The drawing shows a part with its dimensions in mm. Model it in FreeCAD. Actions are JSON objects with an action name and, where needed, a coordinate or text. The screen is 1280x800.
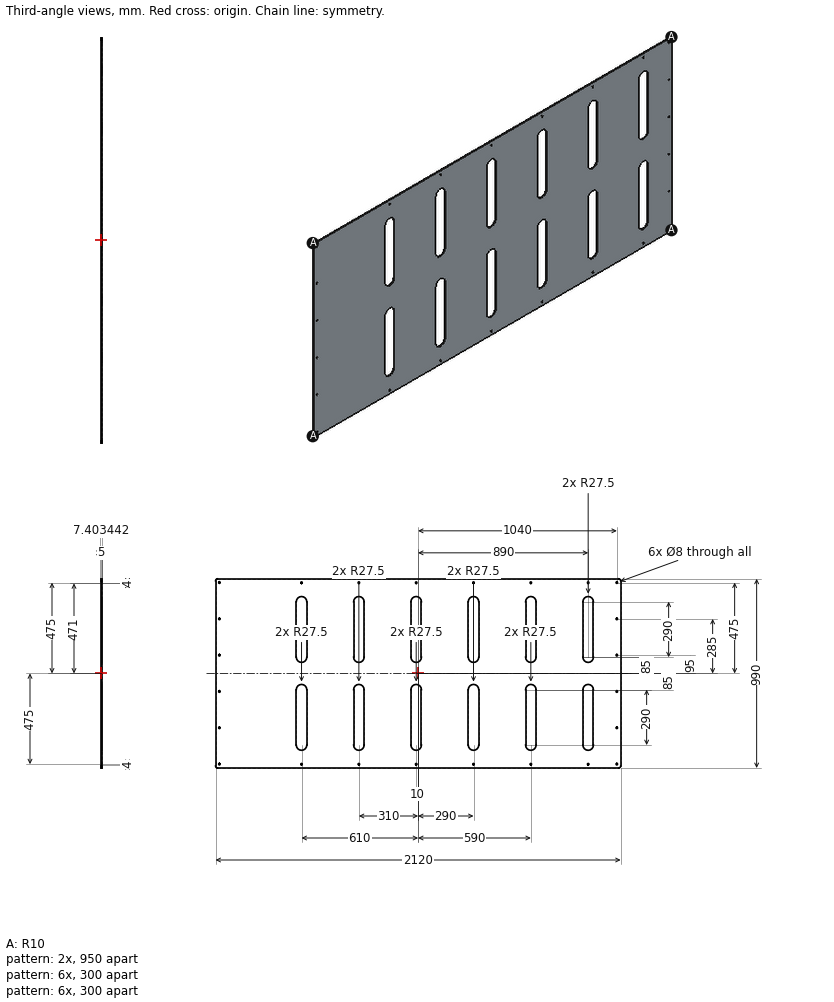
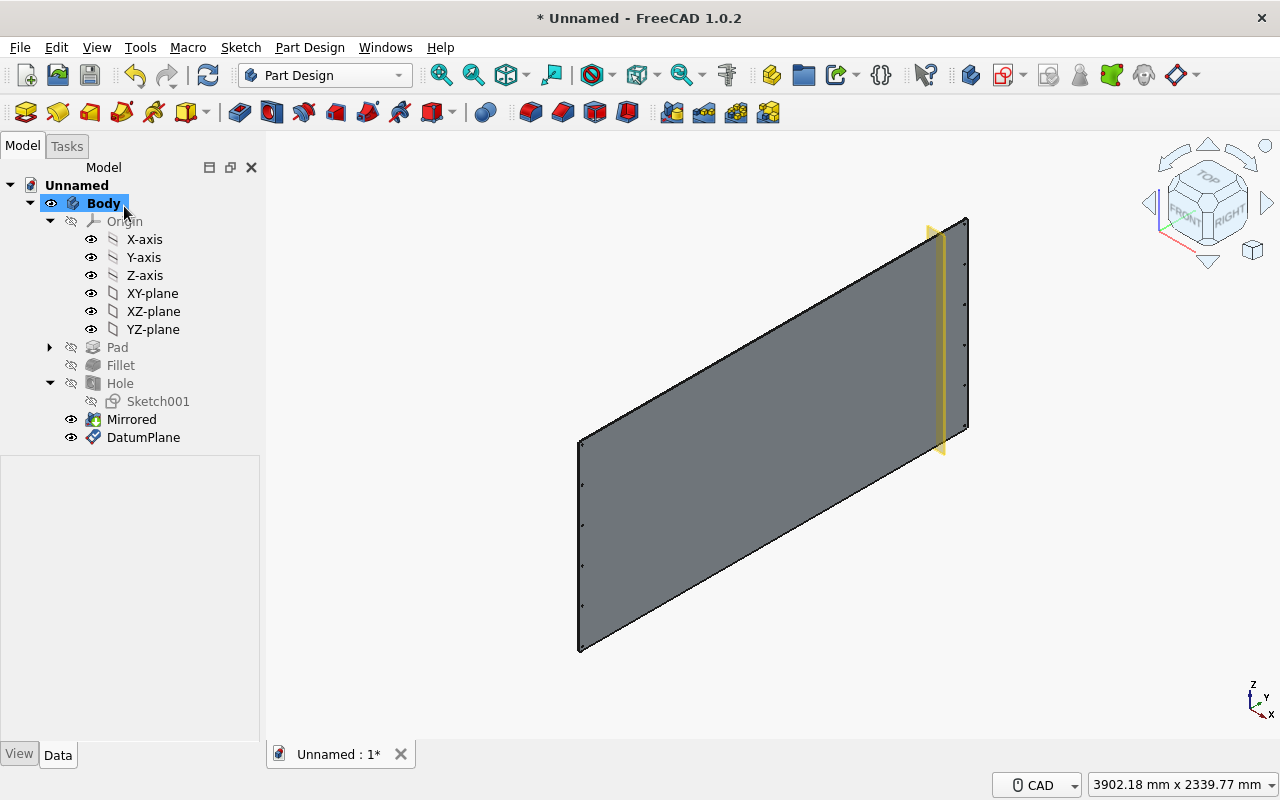
{"action": "left_click", "coordinate": [116, 437]}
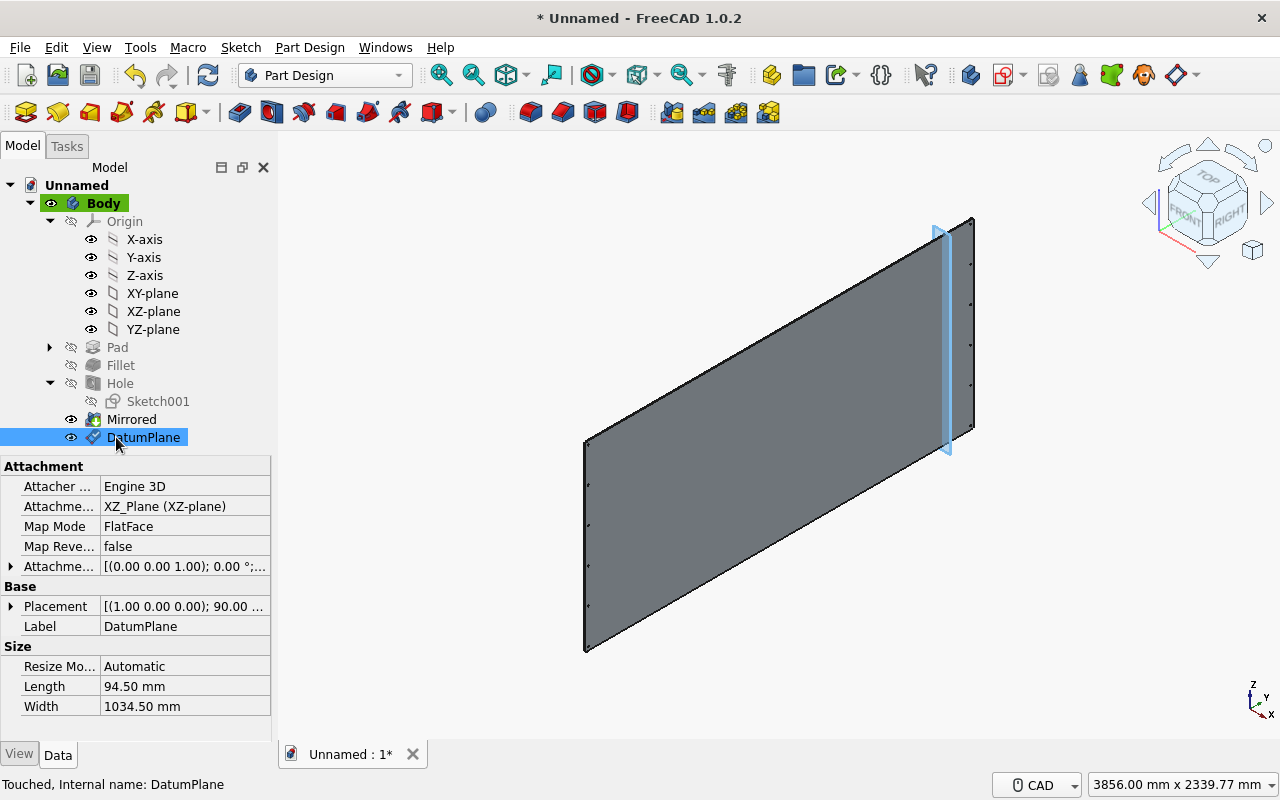
{"action": "left_click", "coordinate": [1004, 76]}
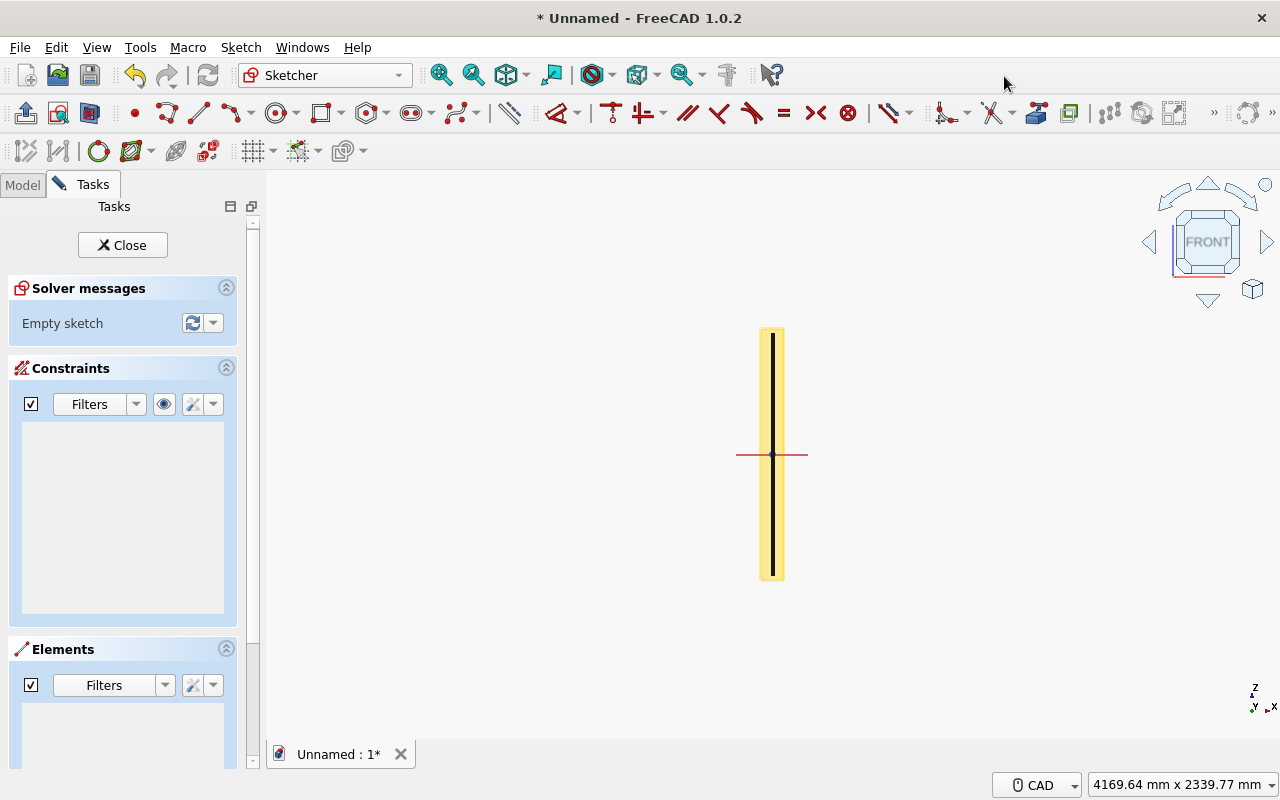
{"action": "left_click", "coordinate": [90, 114]}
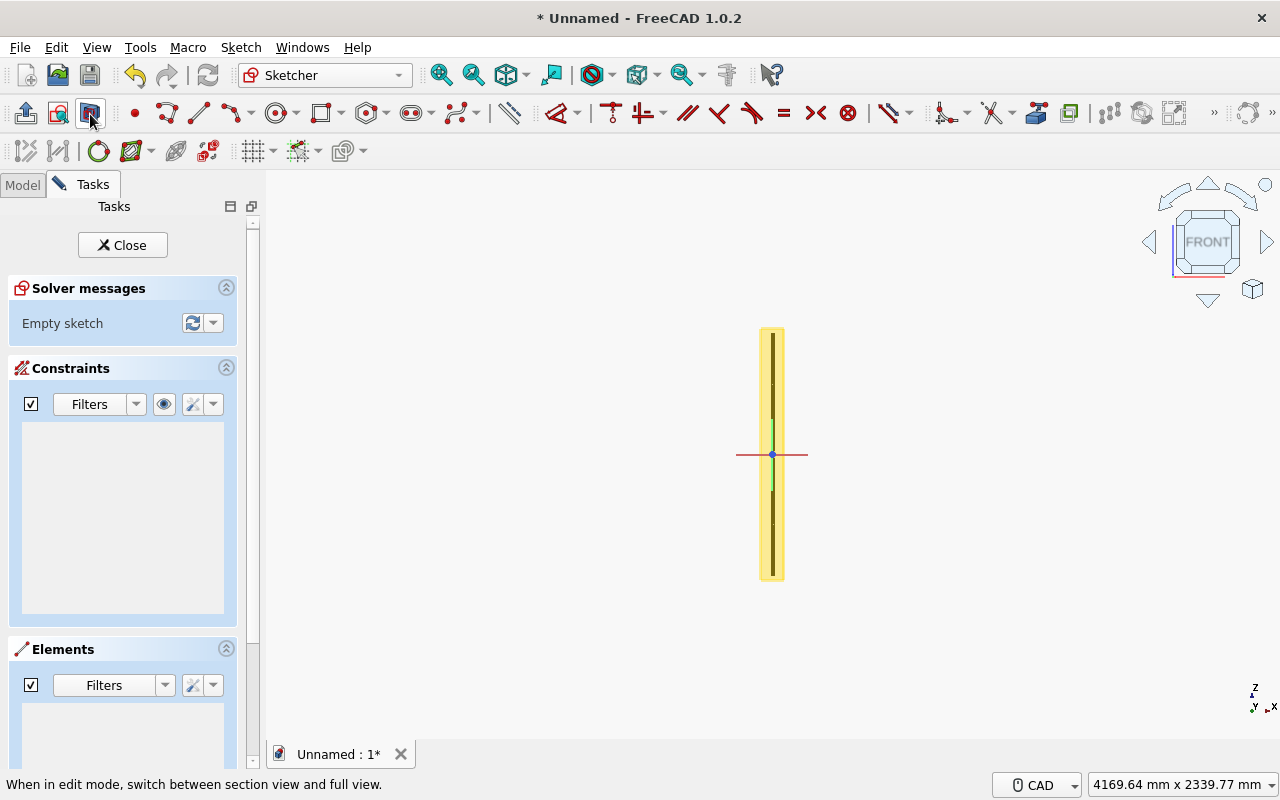
{"action": "scroll", "coordinate": [776, 333], "scroll_direction": "up", "scroll_amount": 15}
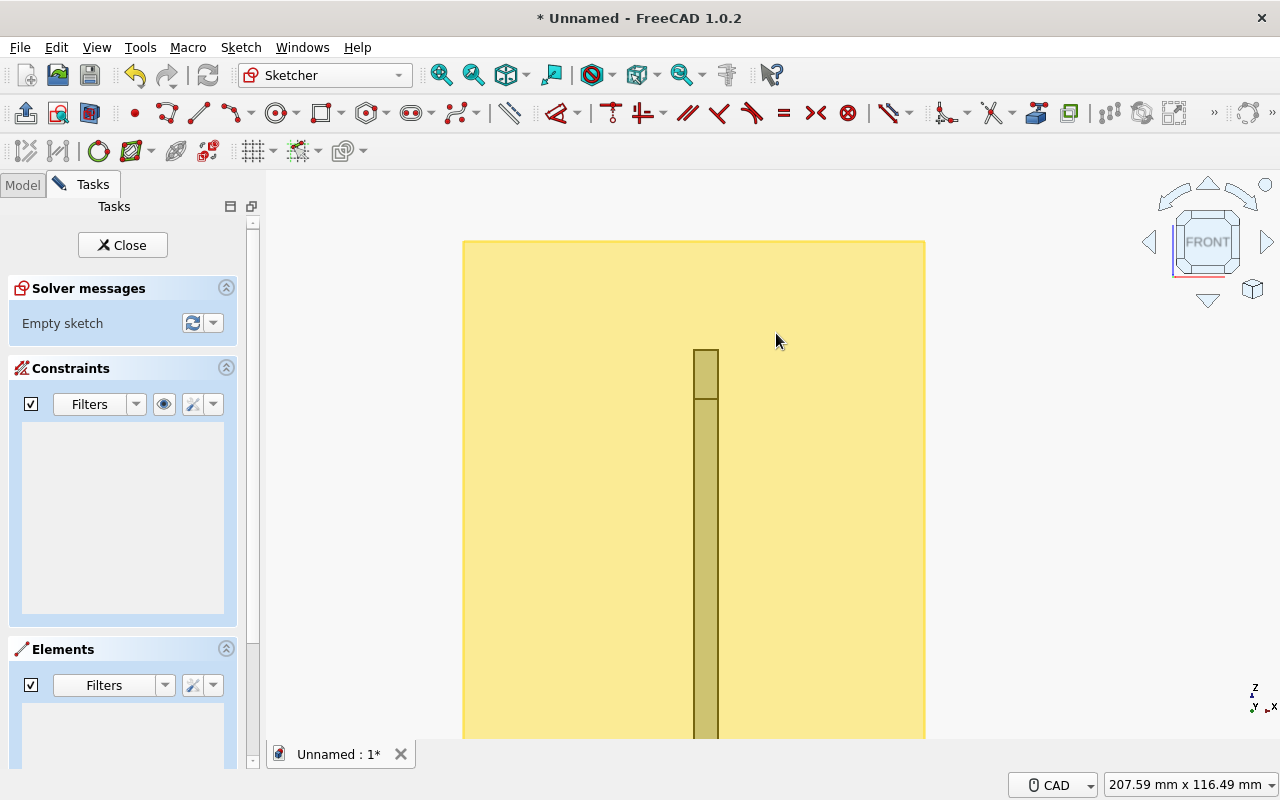
{"action": "scroll", "coordinate": [692, 458], "scroll_direction": "up", "scroll_amount": 12}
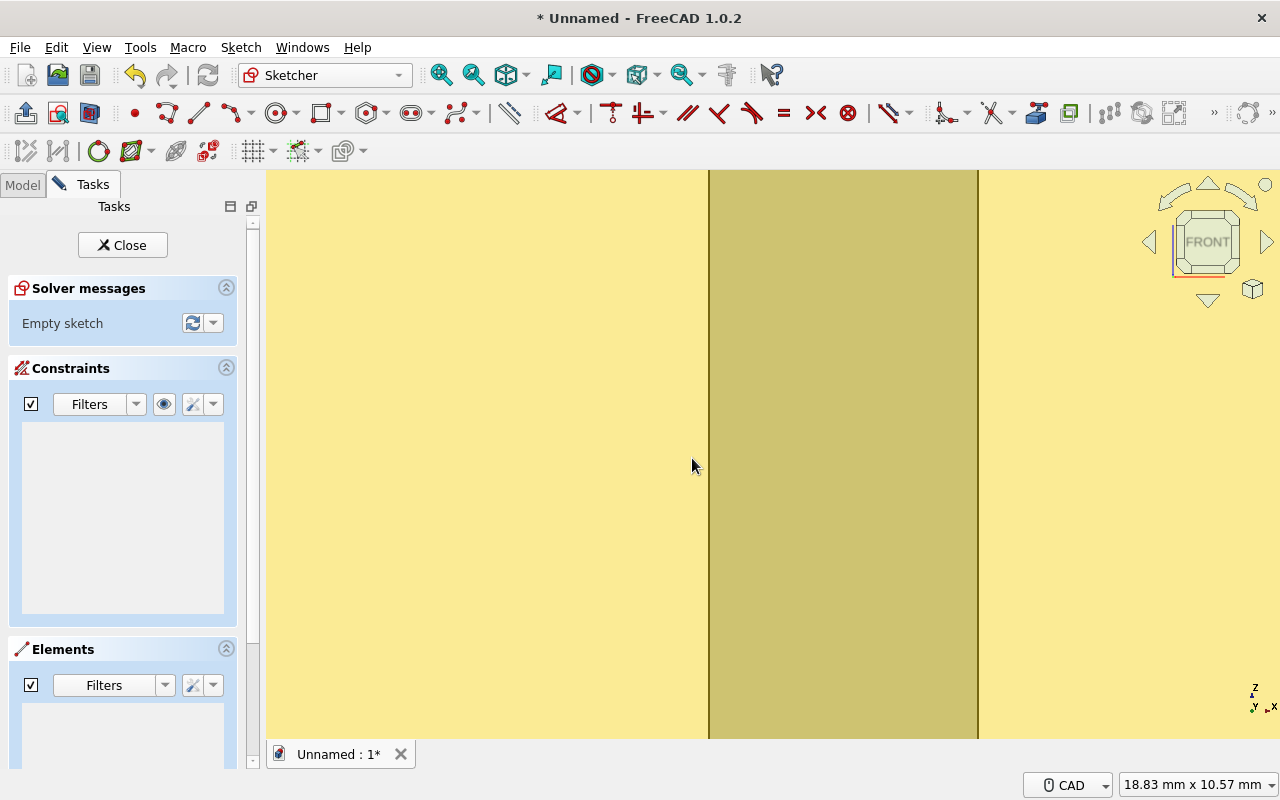
{"action": "left_click", "coordinate": [168, 114]}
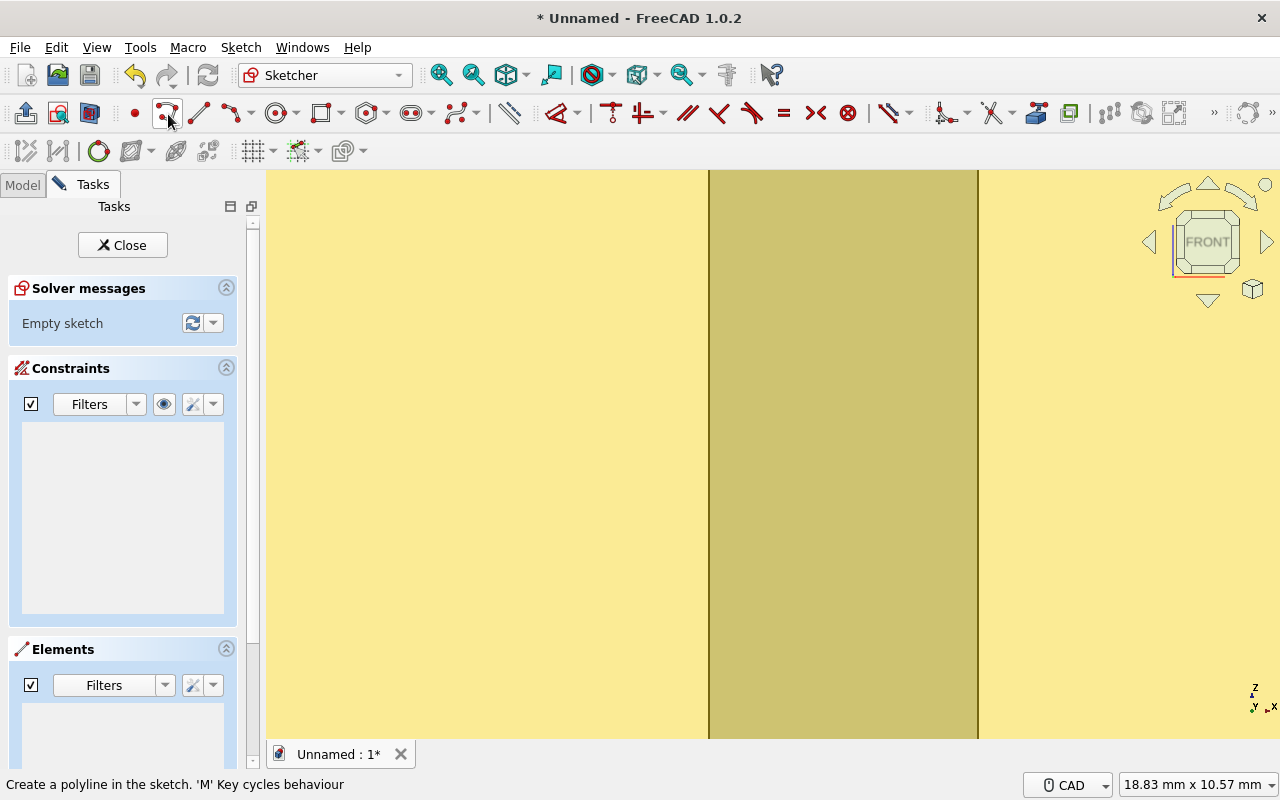
{"action": "left_click", "coordinate": [709, 555]}
{"action": "left_click", "coordinate": [580, 340]}
{"action": "left_click", "coordinate": [978, 340]}
{"action": "left_click", "coordinate": [978, 555]}
{"action": "left_click", "coordinate": [709, 556]}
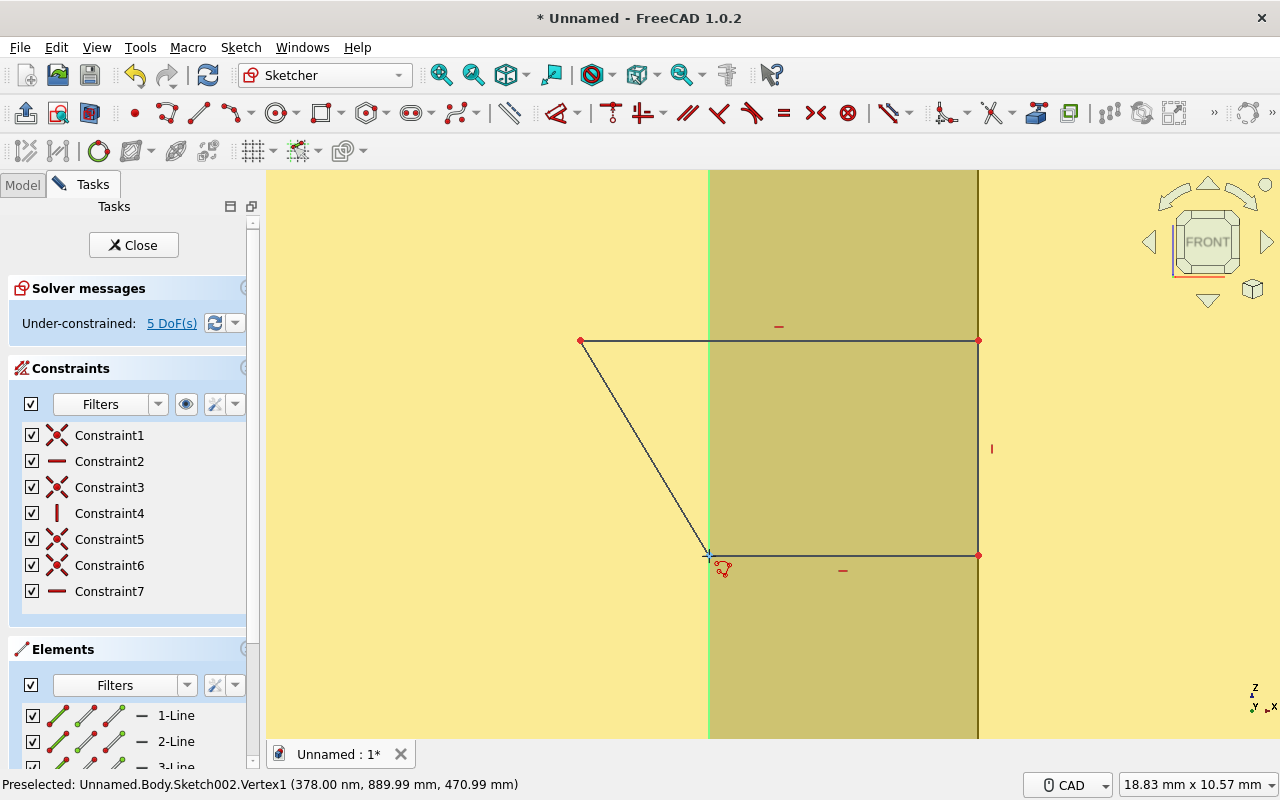
{"action": "left_click", "coordinate": [200, 114]}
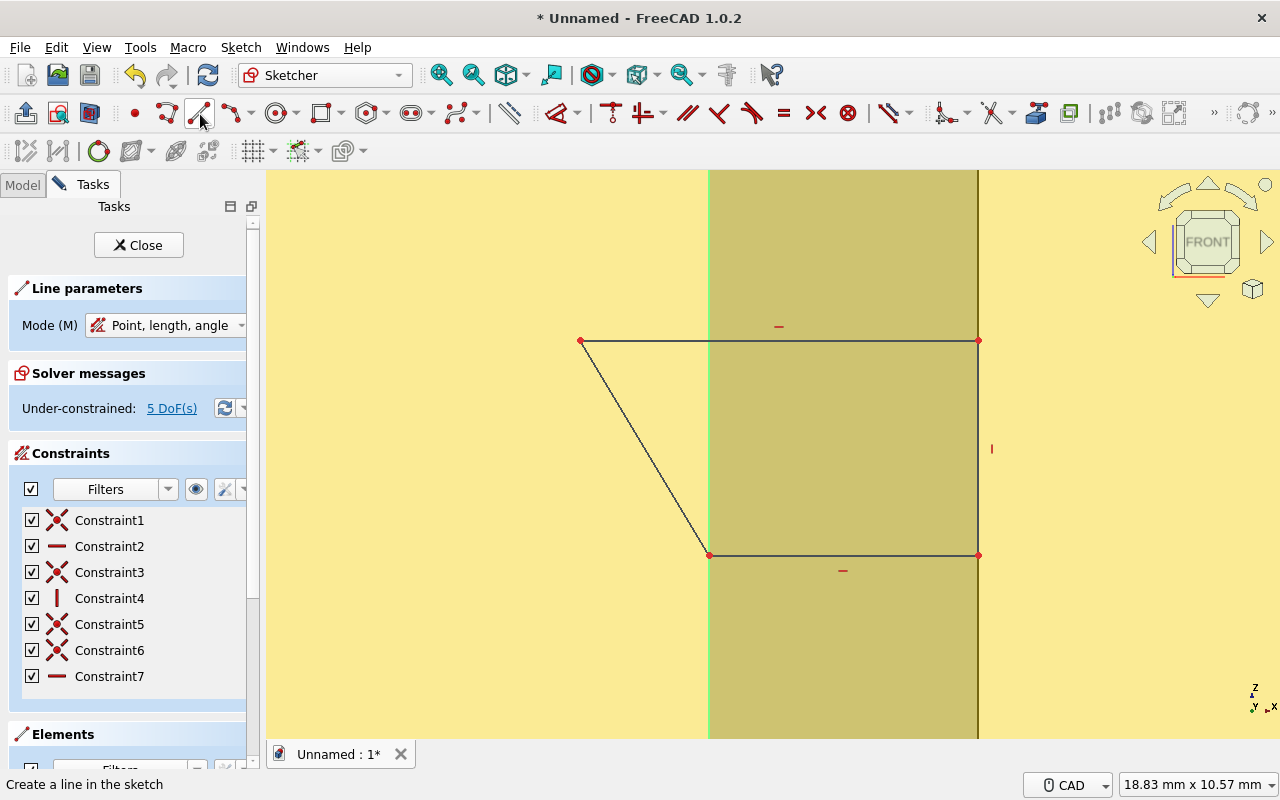
{"action": "left_click", "coordinate": [540, 340]}
{"action": "left_click", "coordinate": [420, 340]}
{"action": "key", "text": "Escape"}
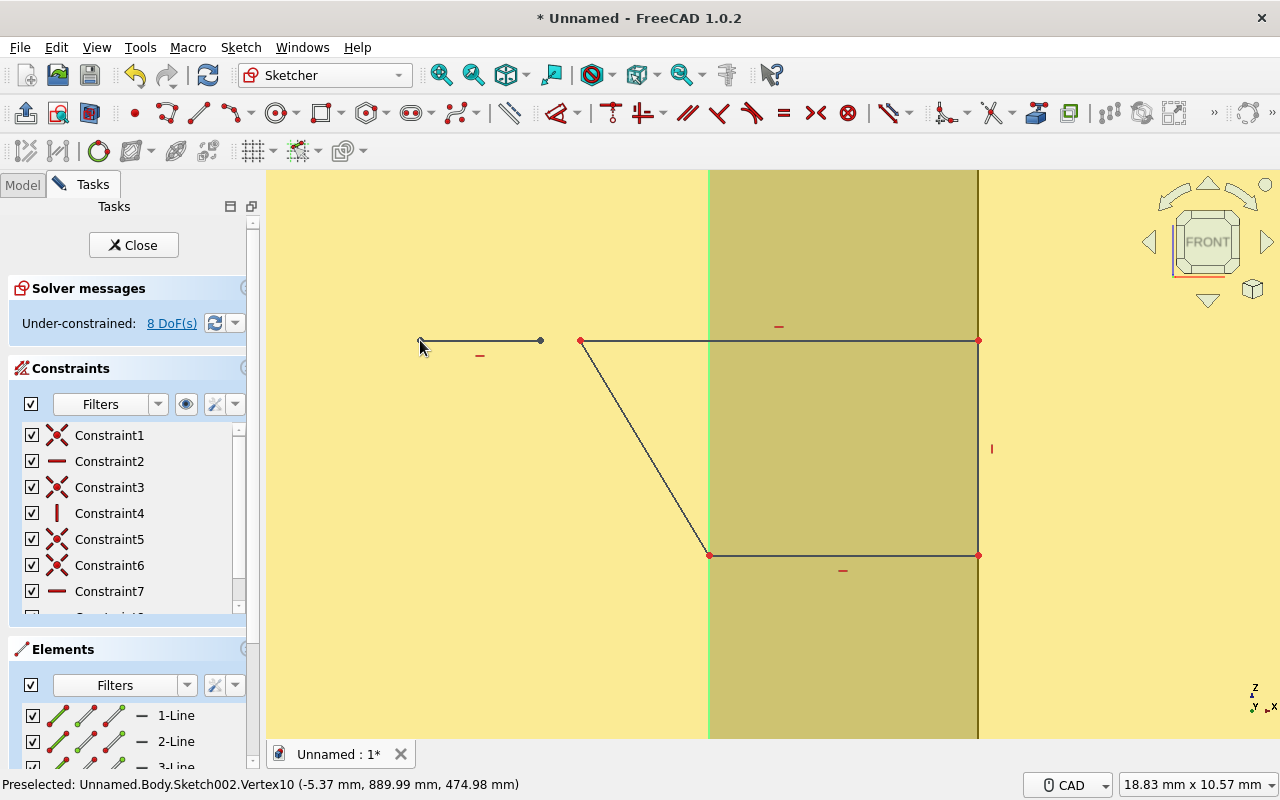
{"action": "left_click", "coordinate": [504, 341]}